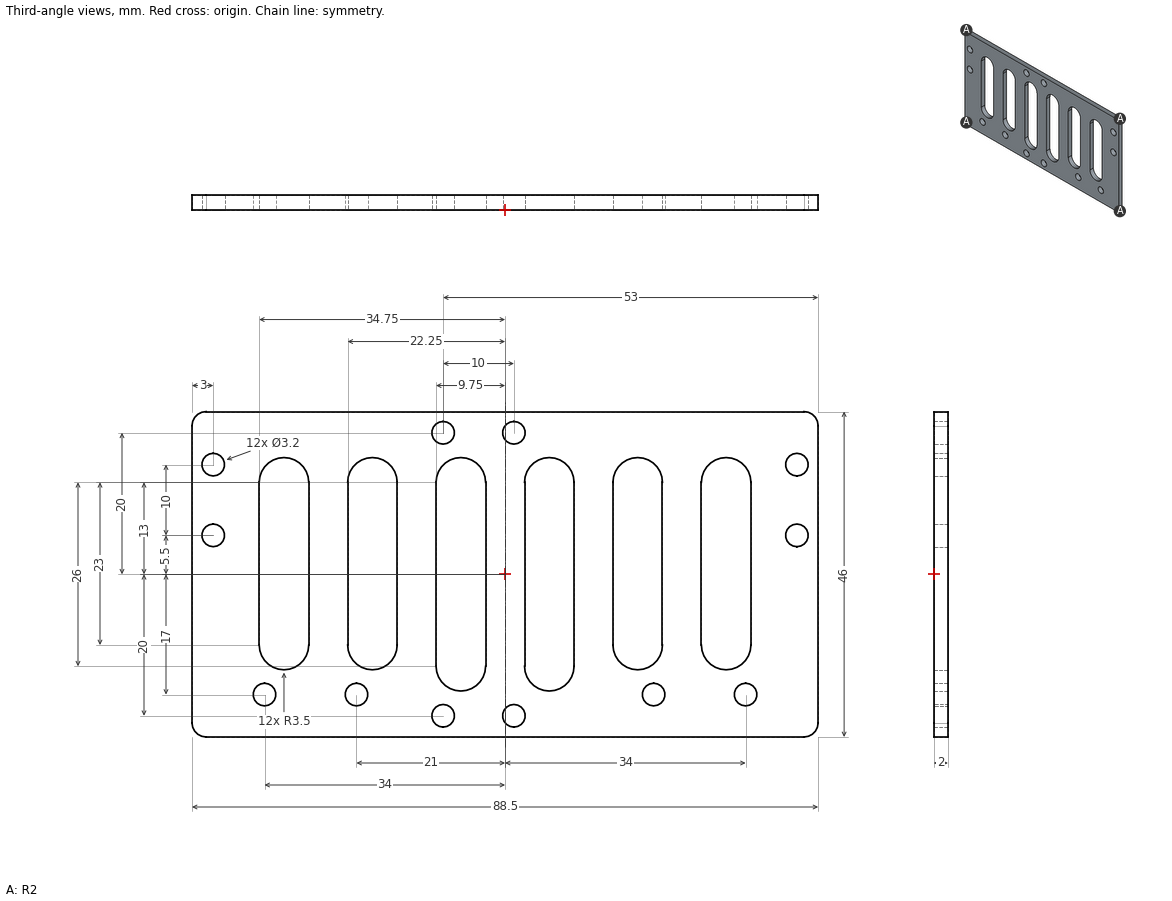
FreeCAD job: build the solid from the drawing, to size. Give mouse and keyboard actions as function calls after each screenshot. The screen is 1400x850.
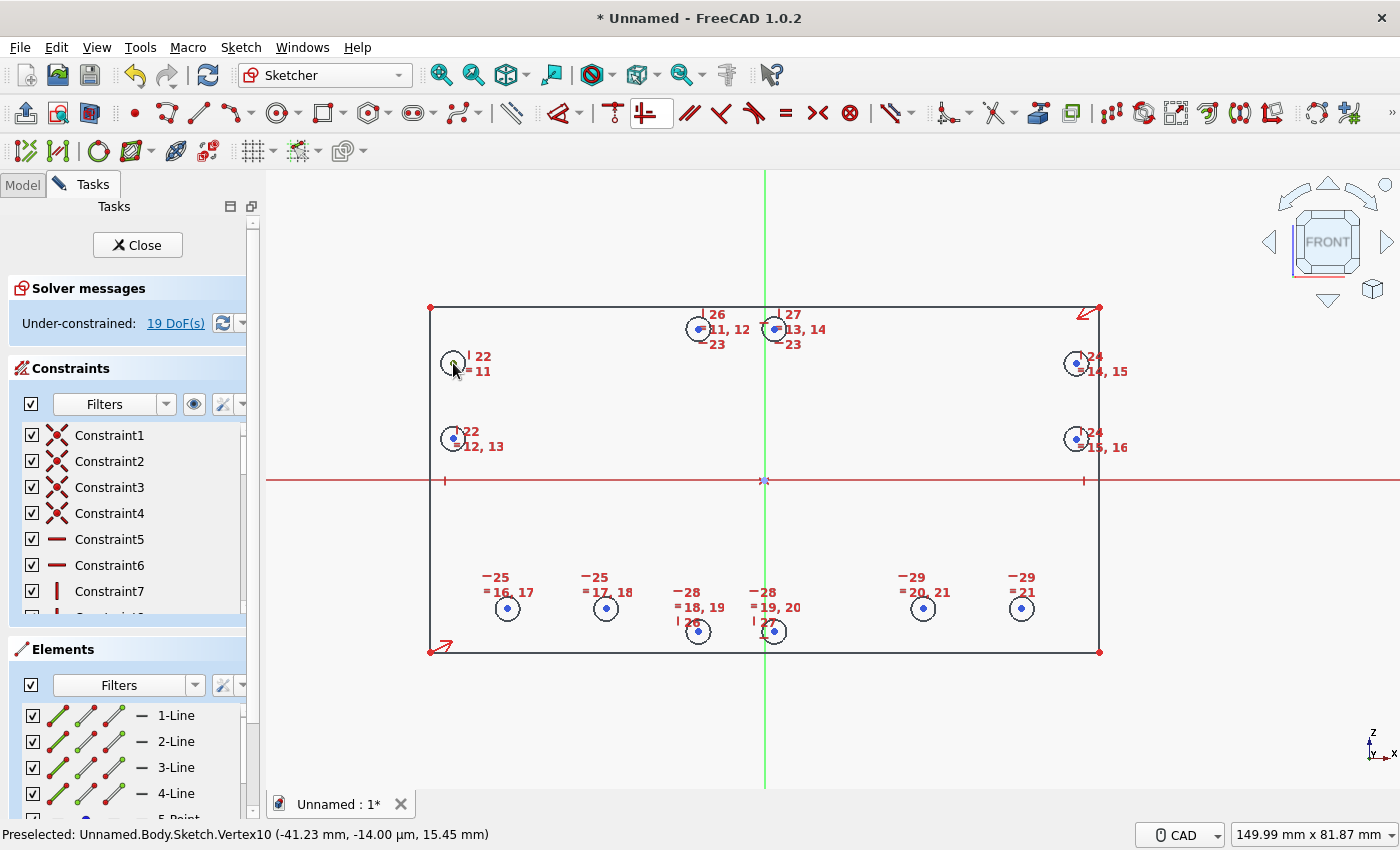
click(1076, 364)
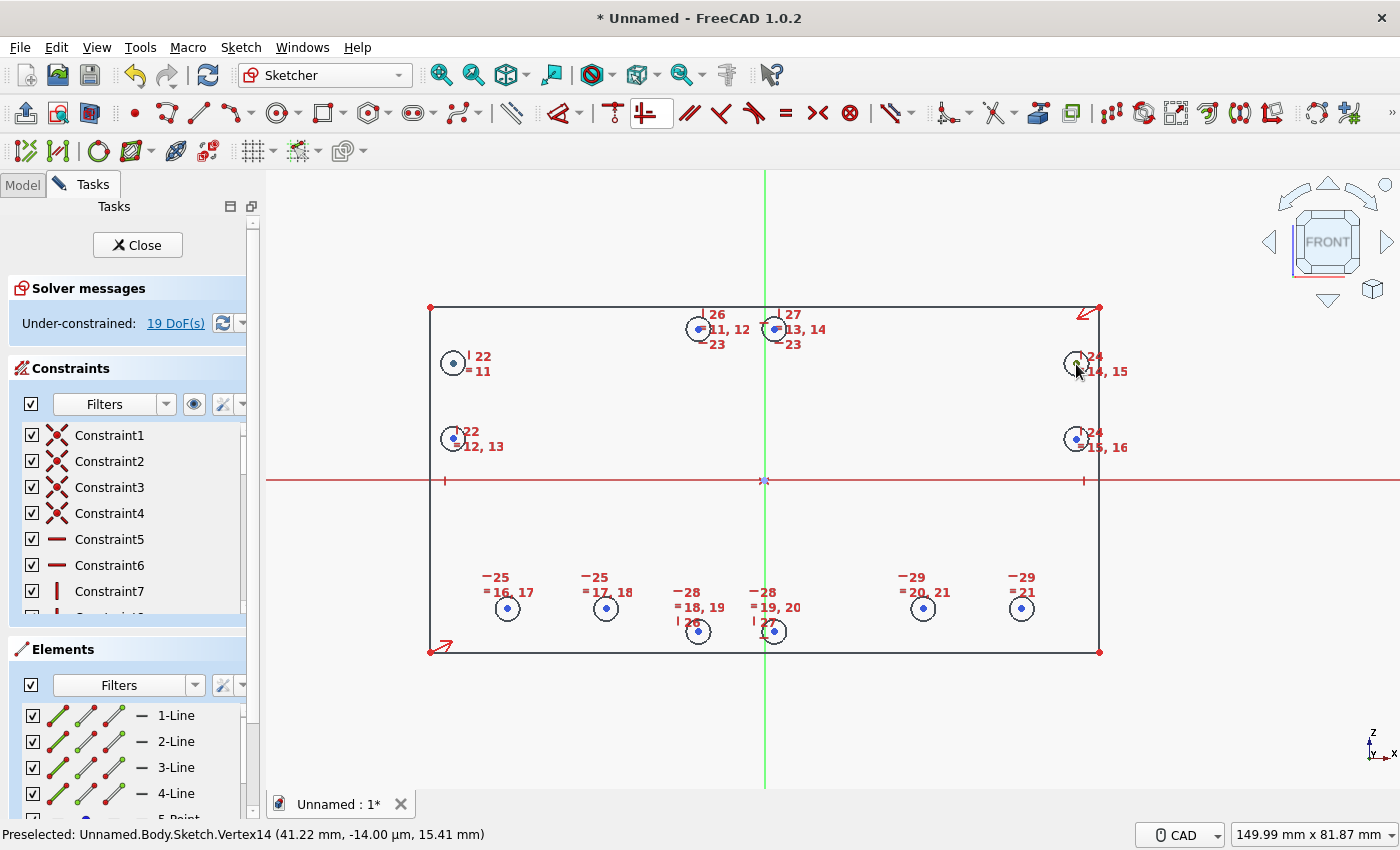
click(765, 721)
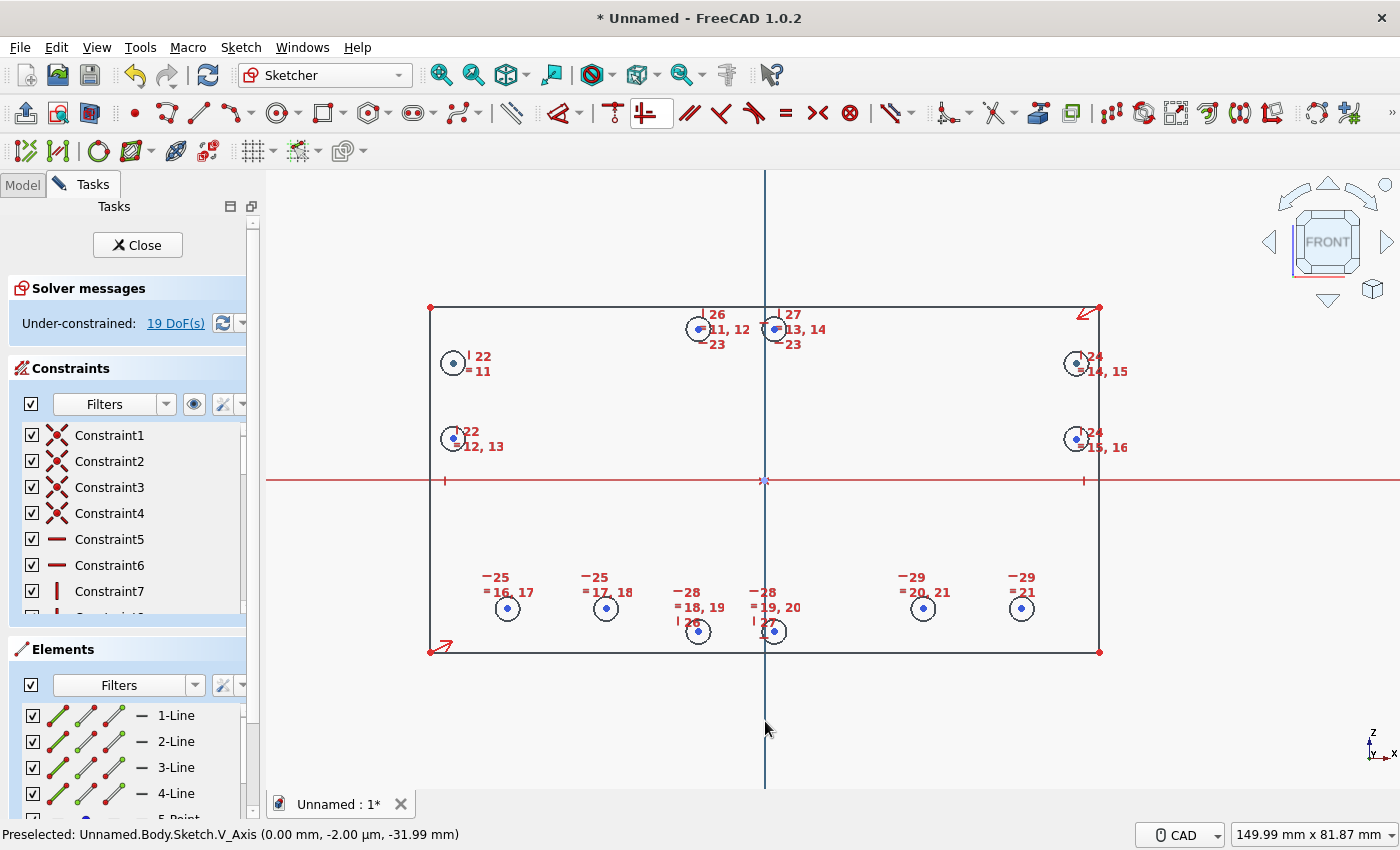
click(818, 114)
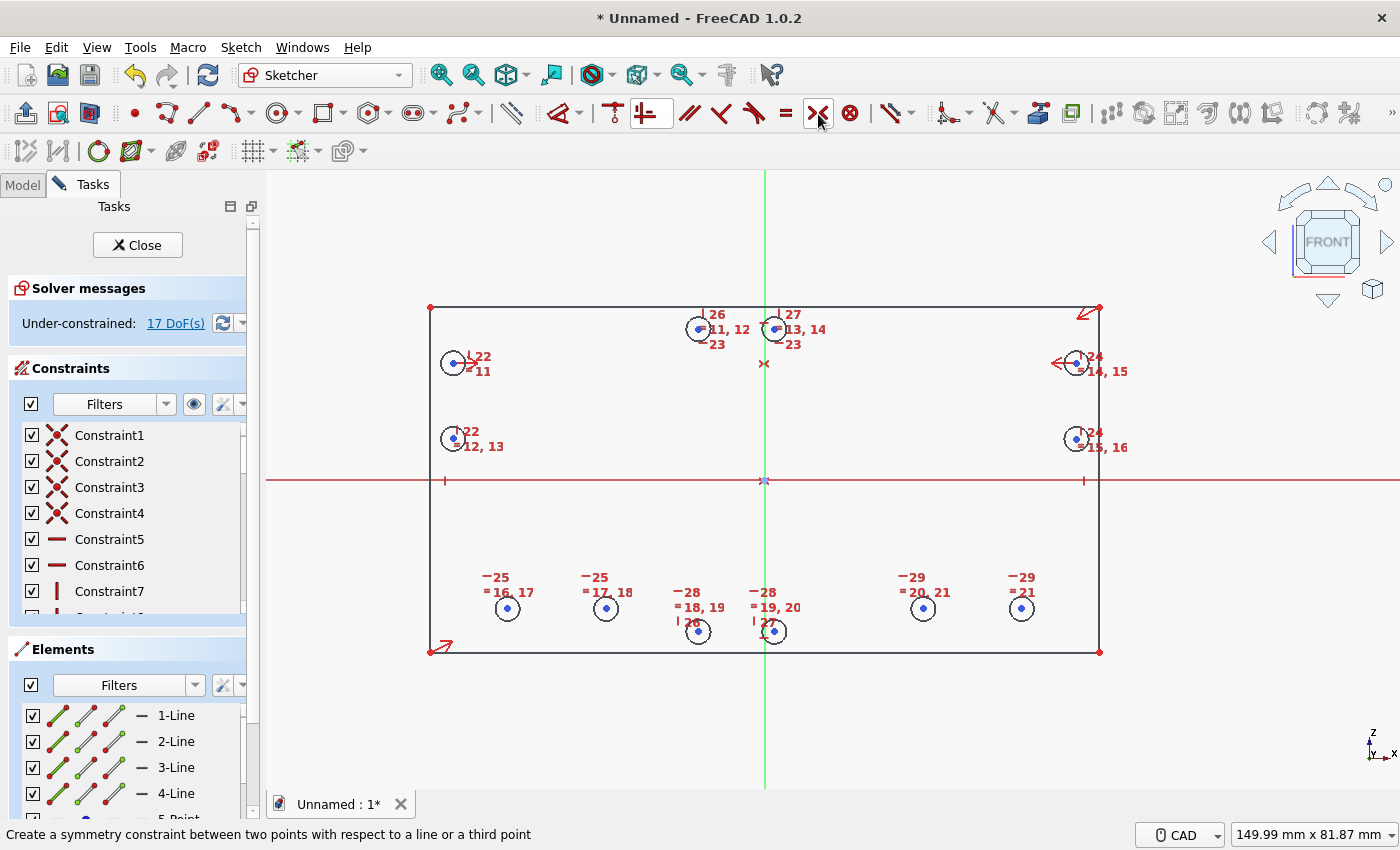
click(606, 609)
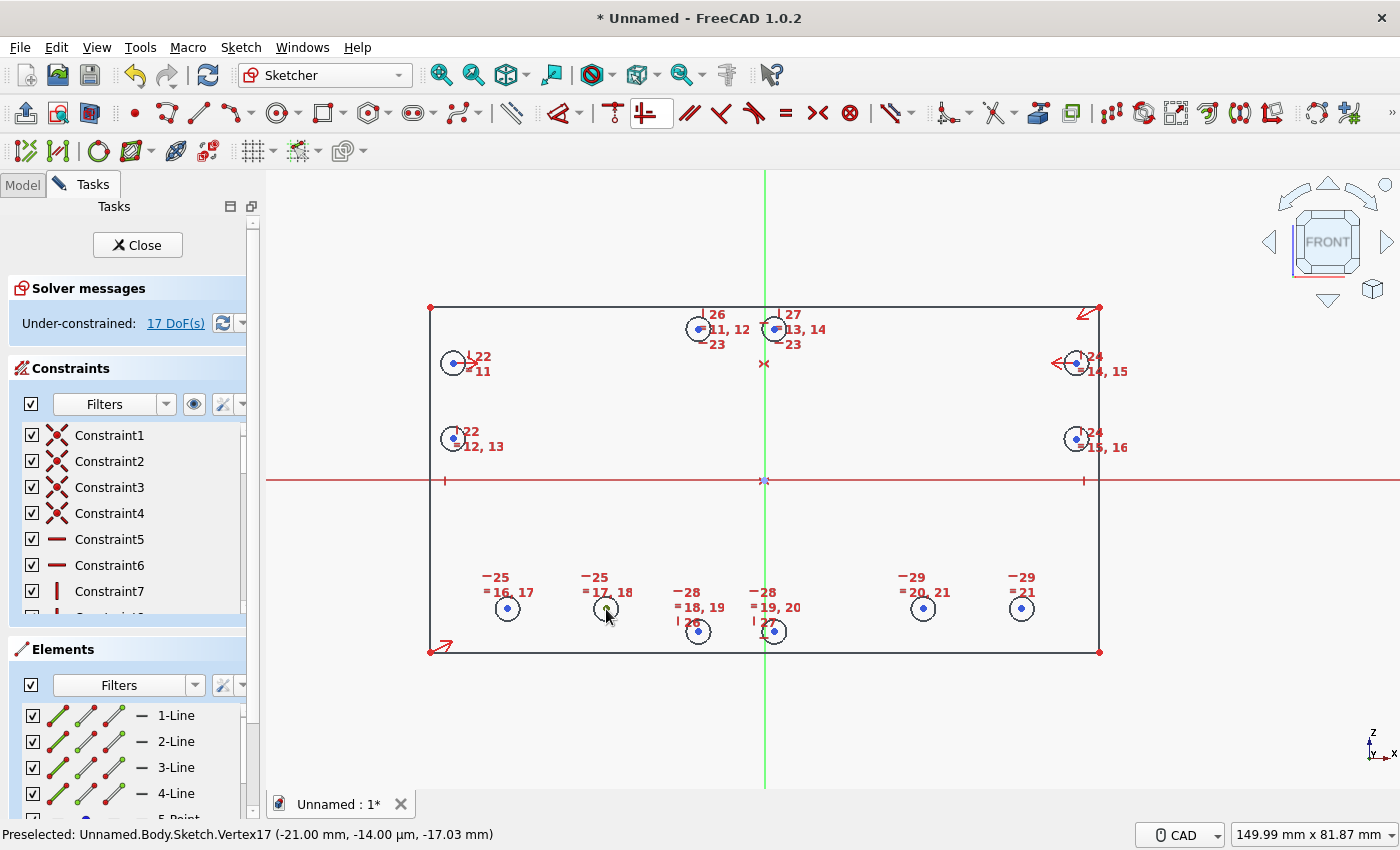
click(923, 609)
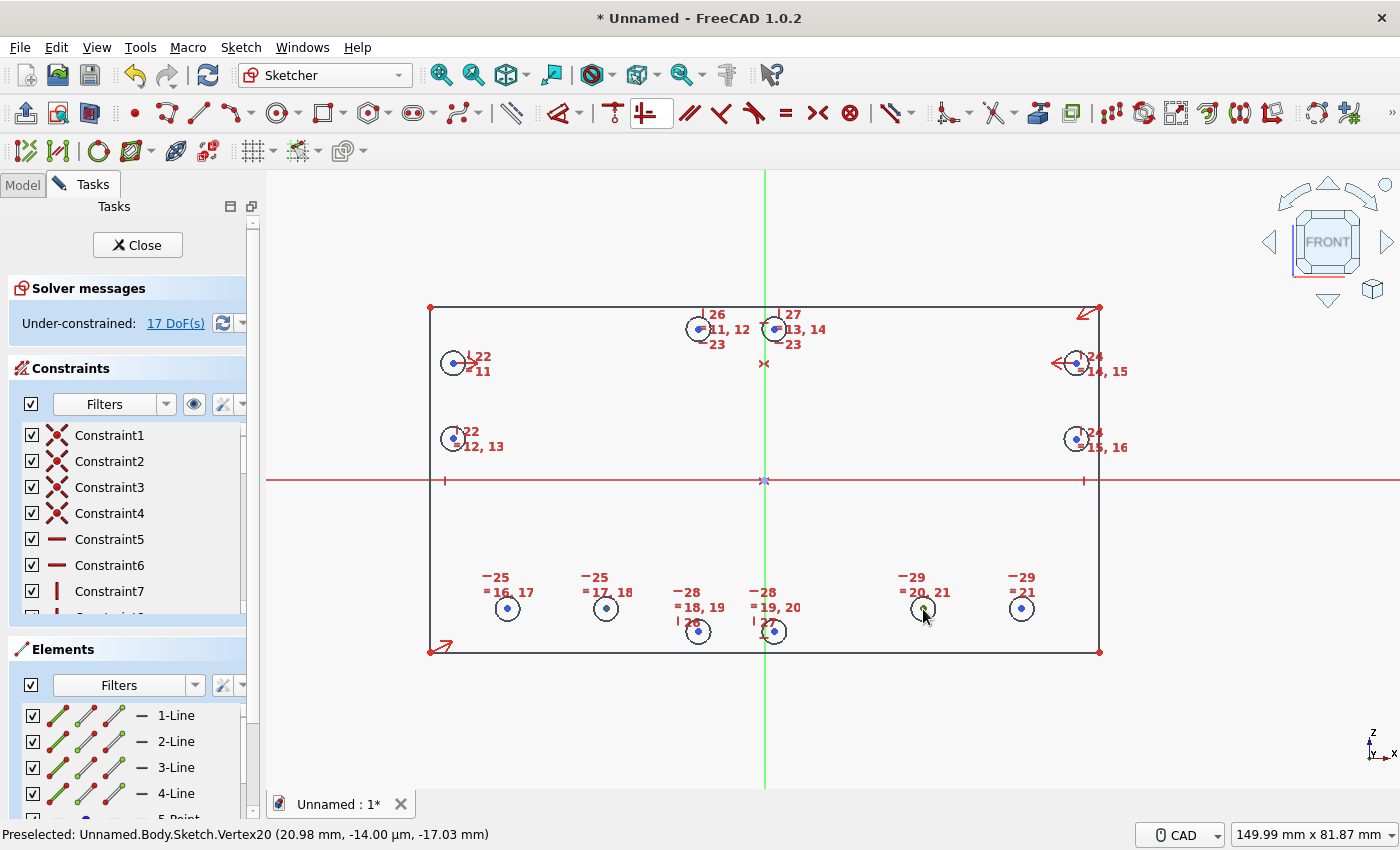
click(765, 721)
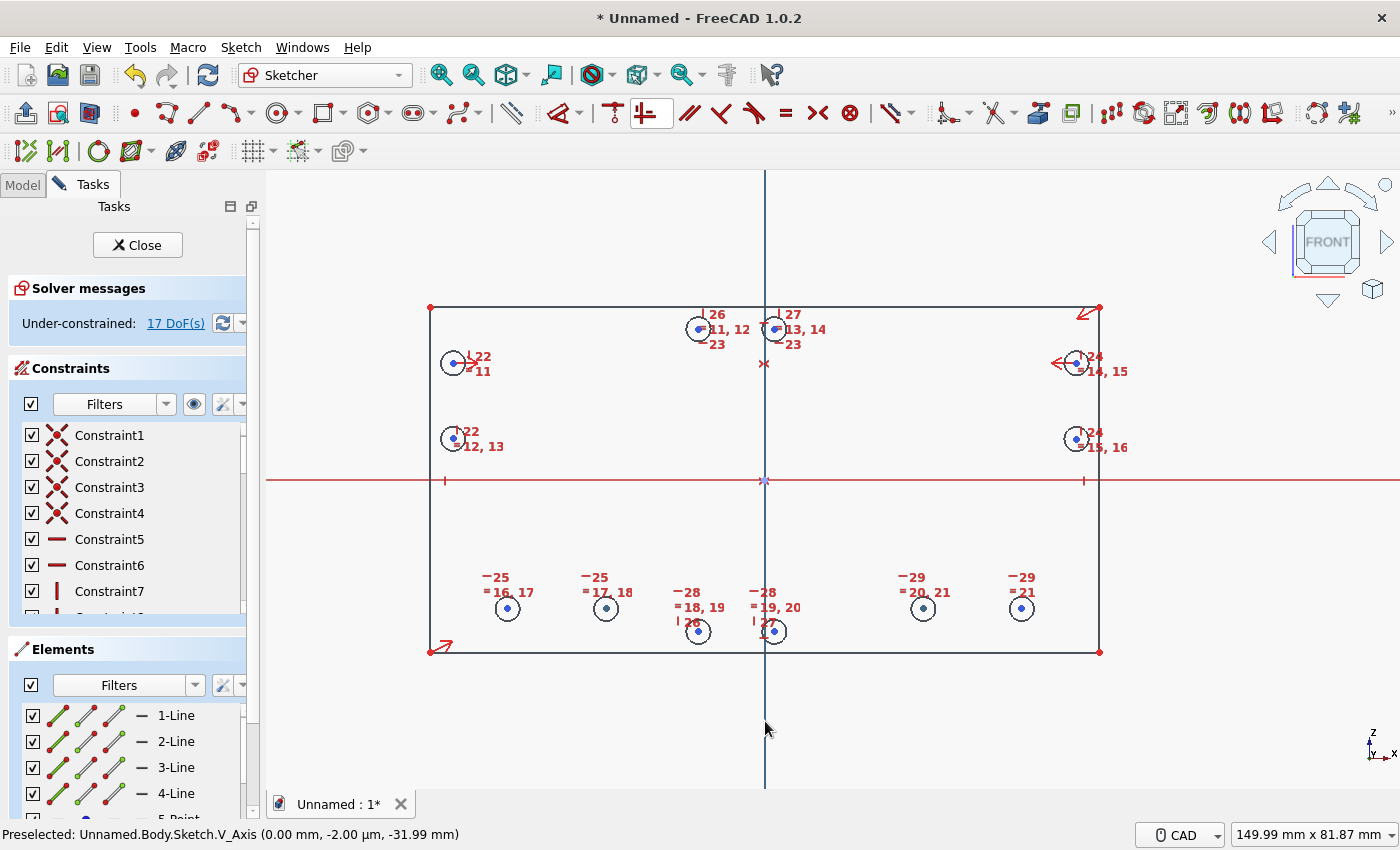
click(818, 114)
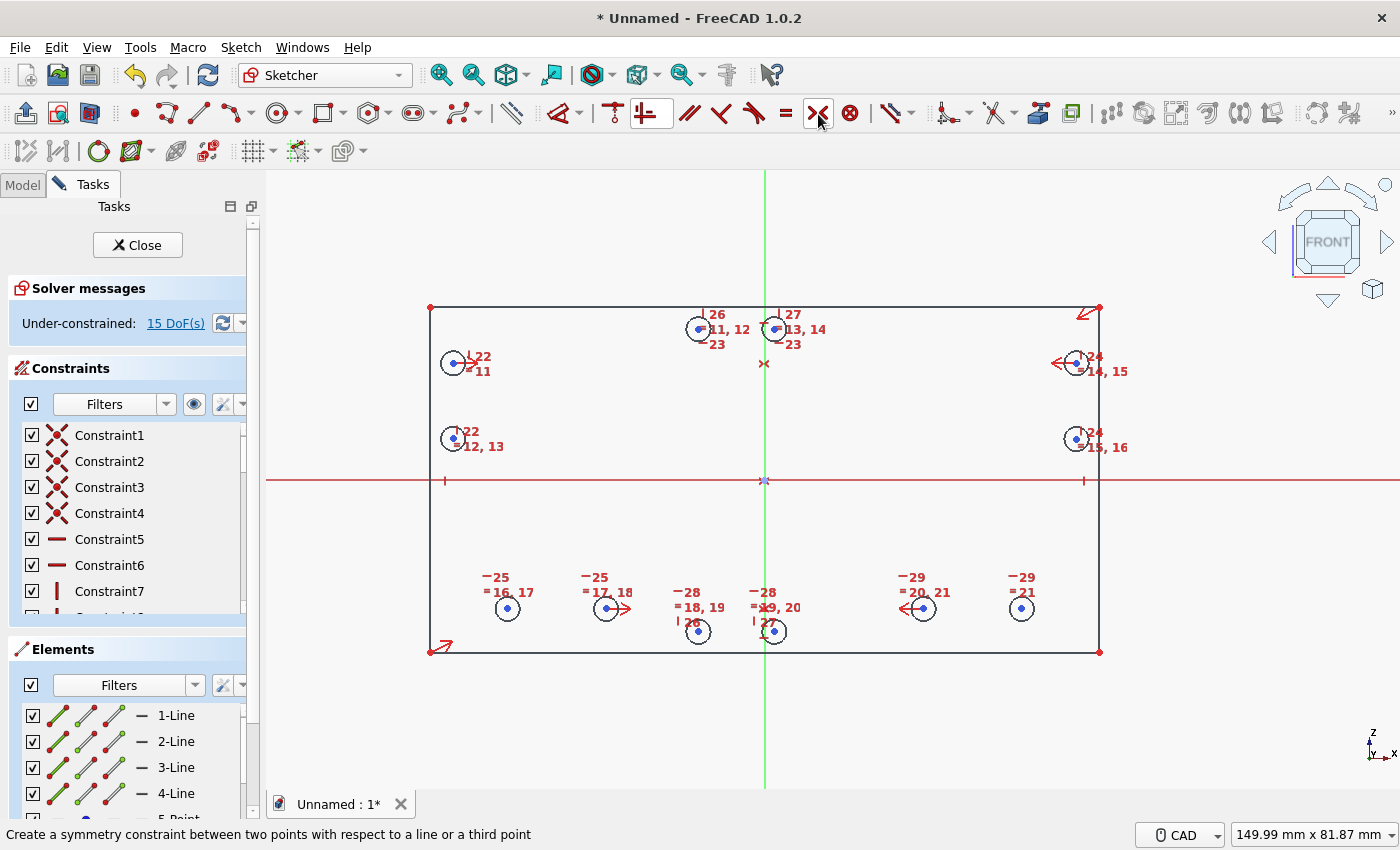
click(558, 114)